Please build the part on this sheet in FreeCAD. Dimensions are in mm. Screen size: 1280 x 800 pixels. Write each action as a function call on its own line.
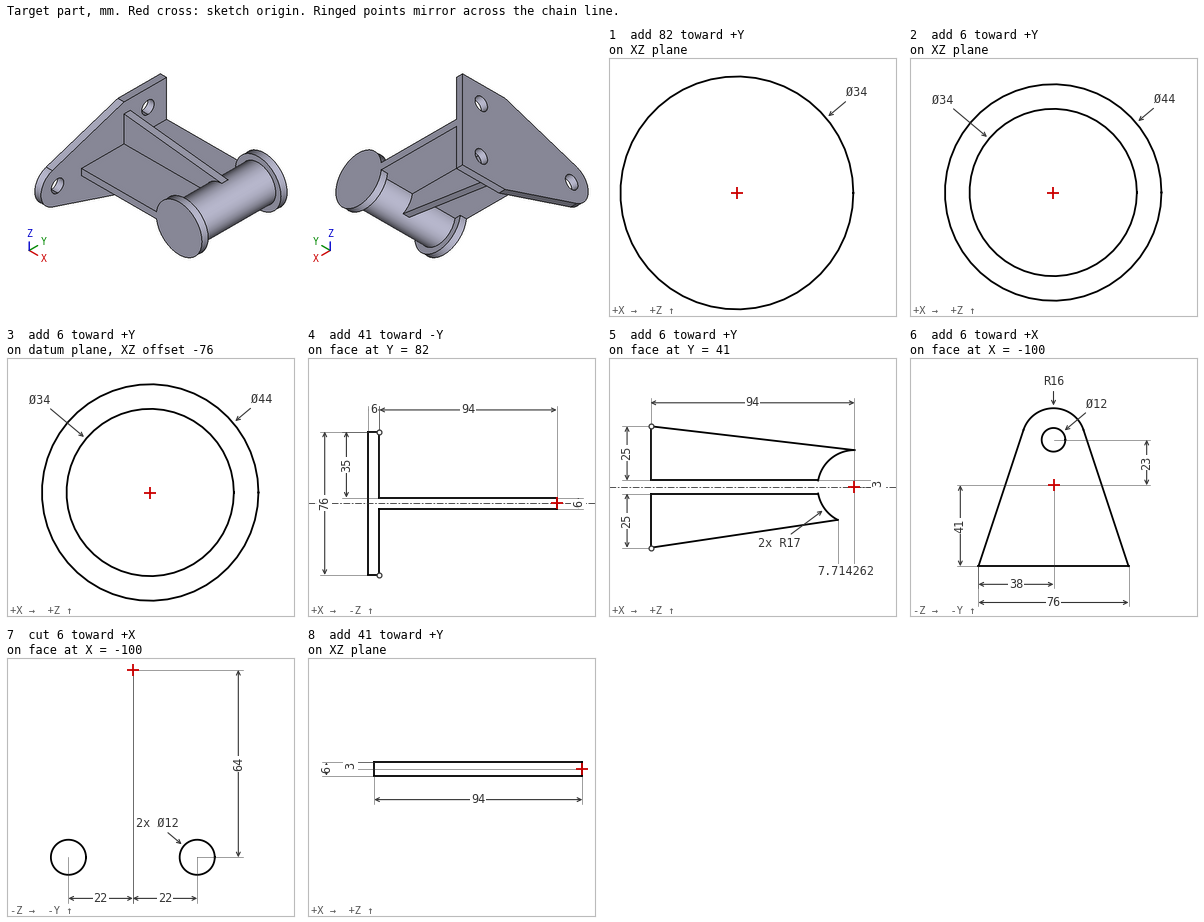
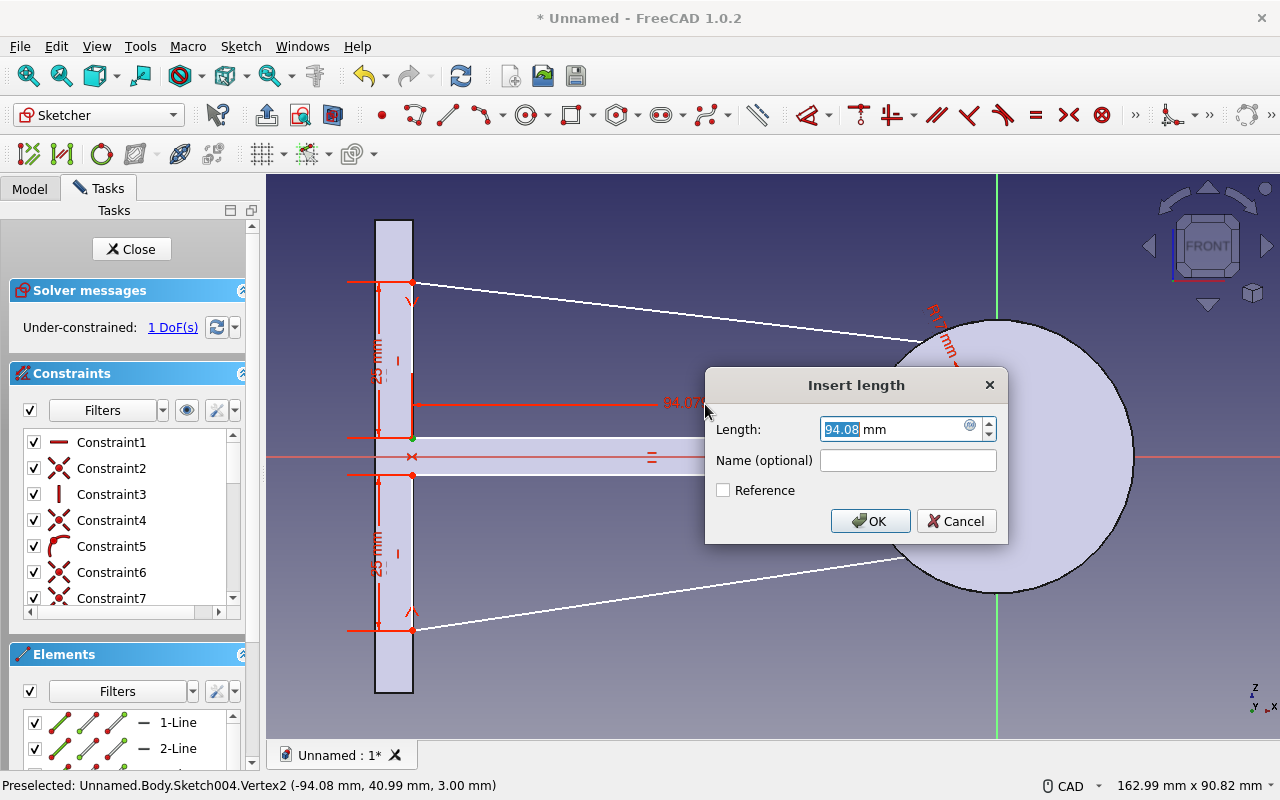
text(94)
key(Return)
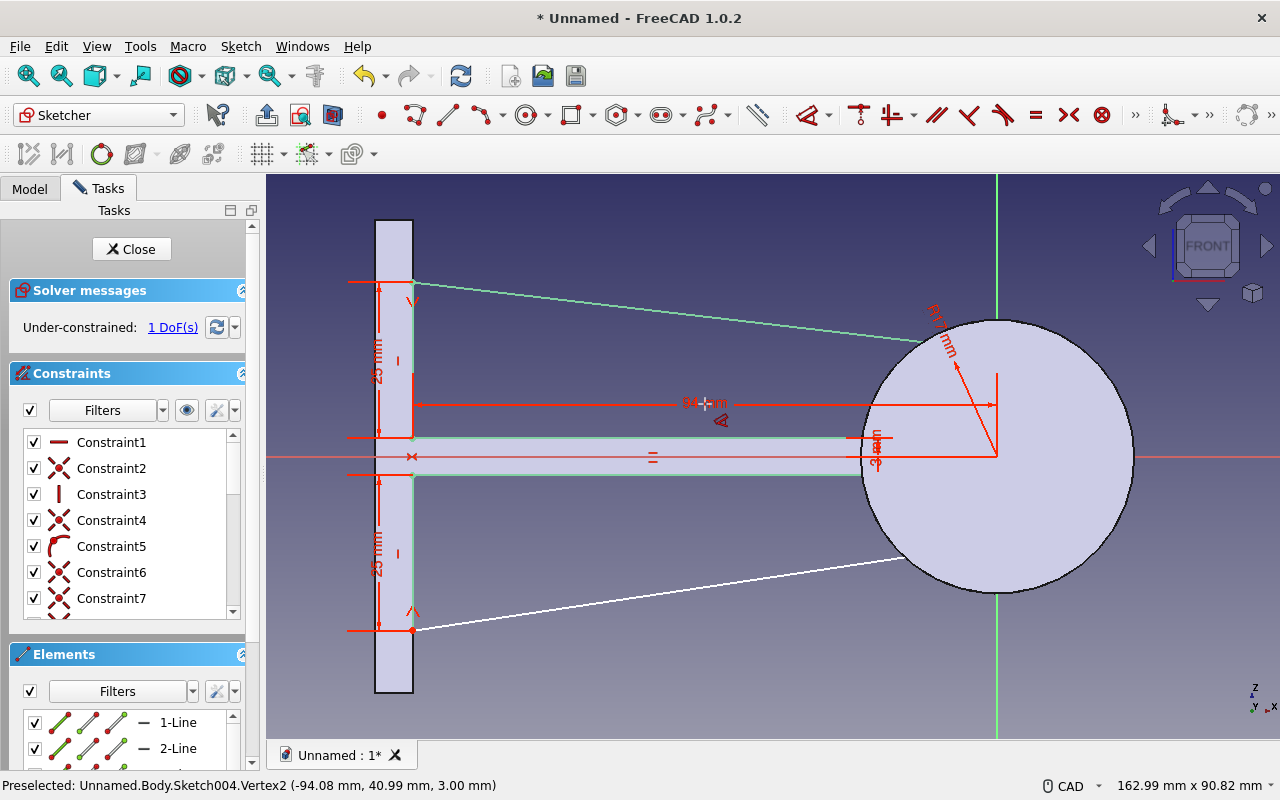
click(949, 551)
click(973, 585)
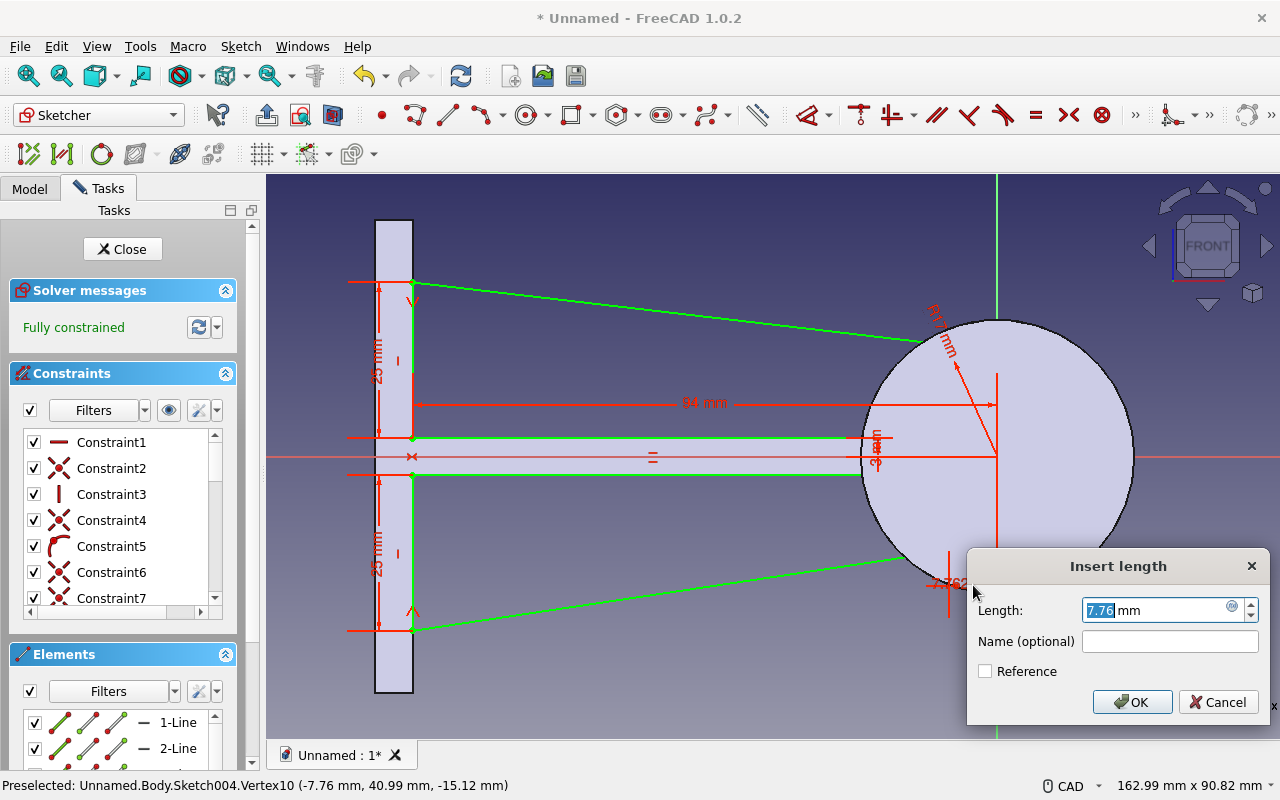
text(7.714262)
key(Return)
key(Escape)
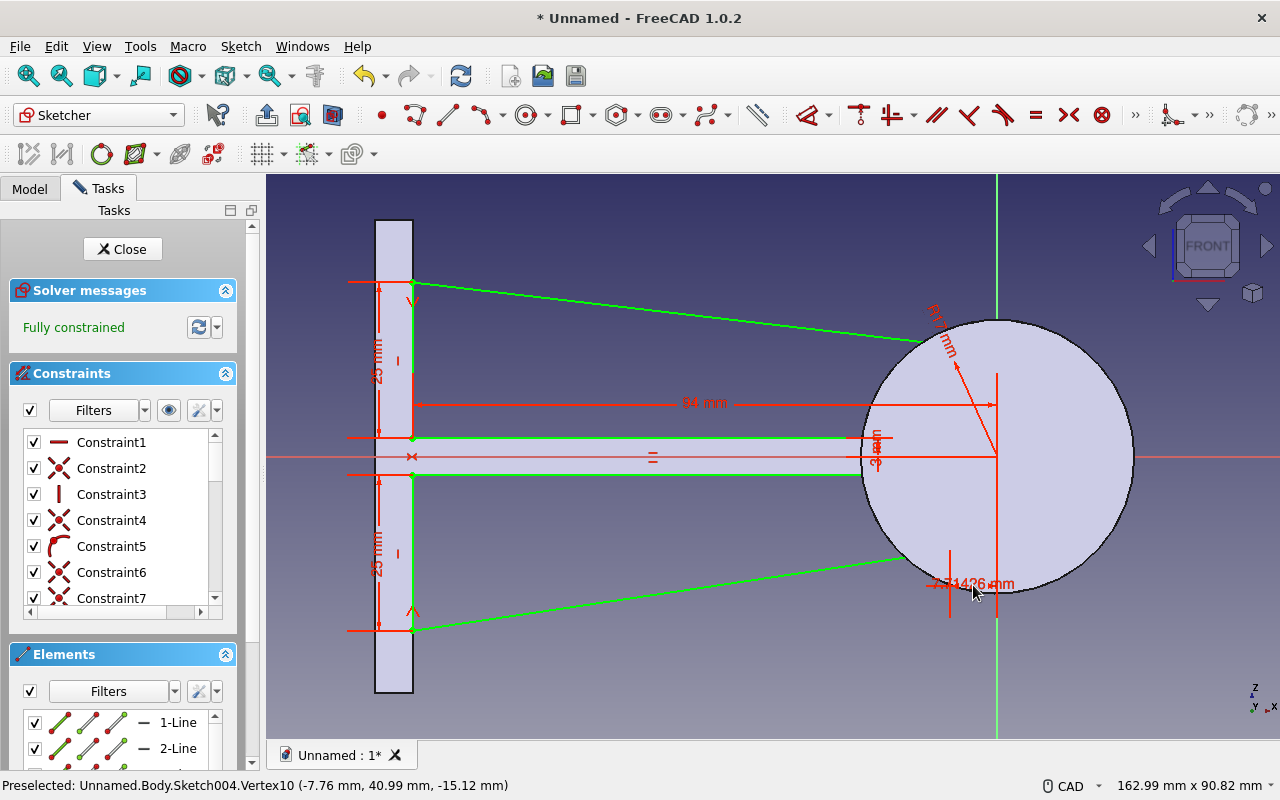
click(123, 249)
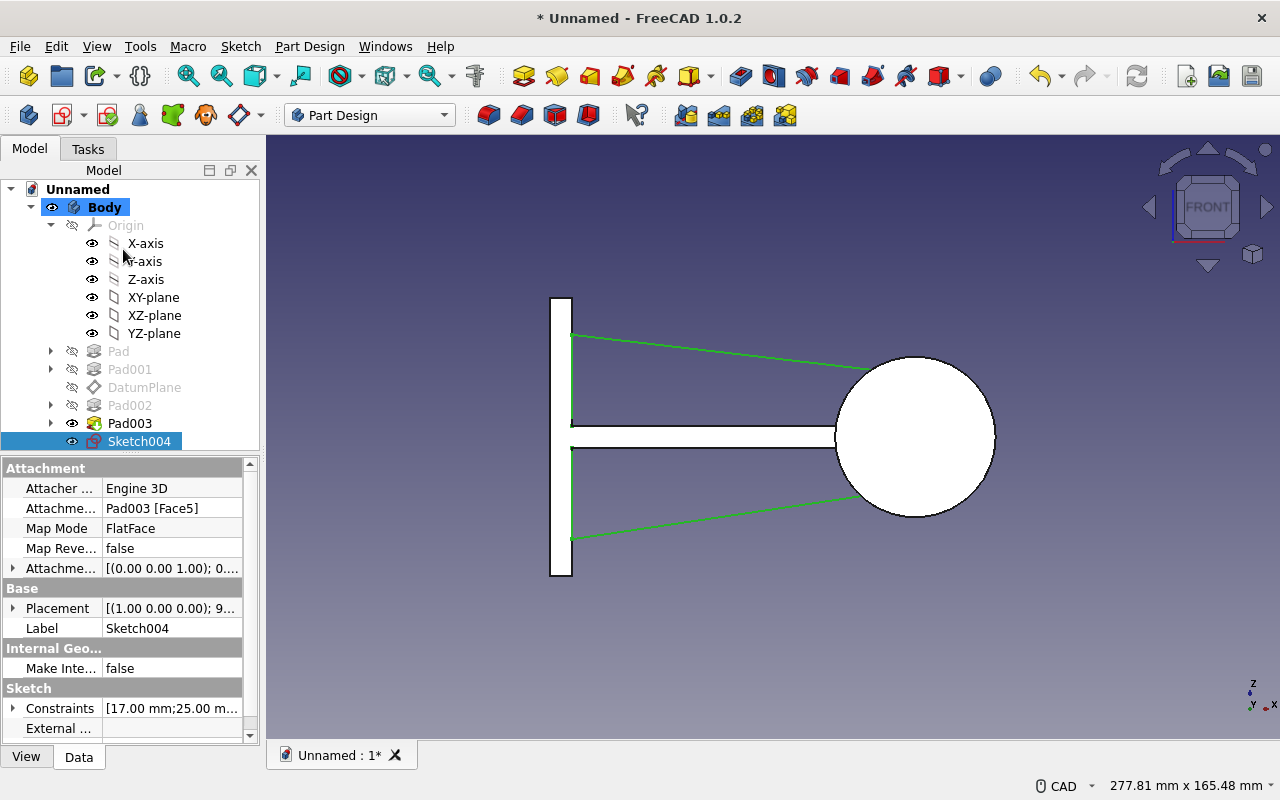
click(524, 76)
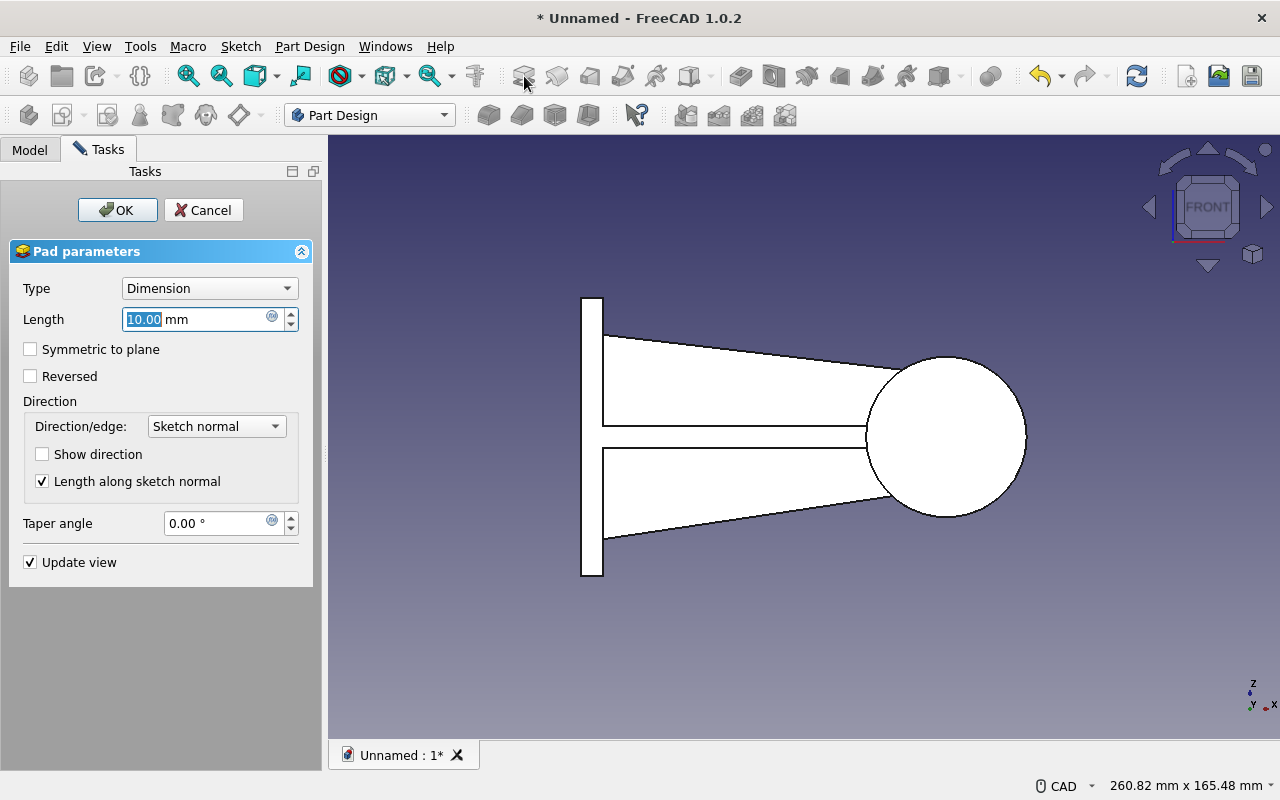
text(6)
key(Tab)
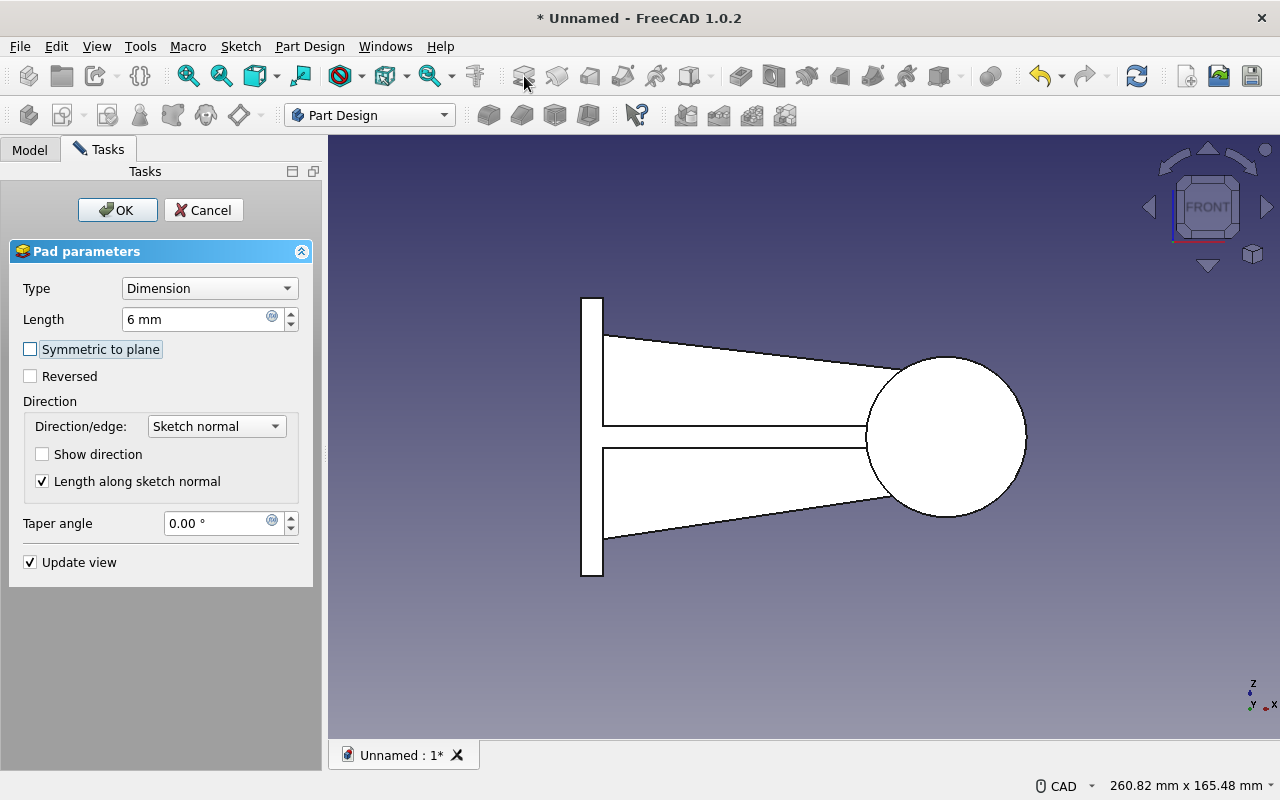
click(31, 376)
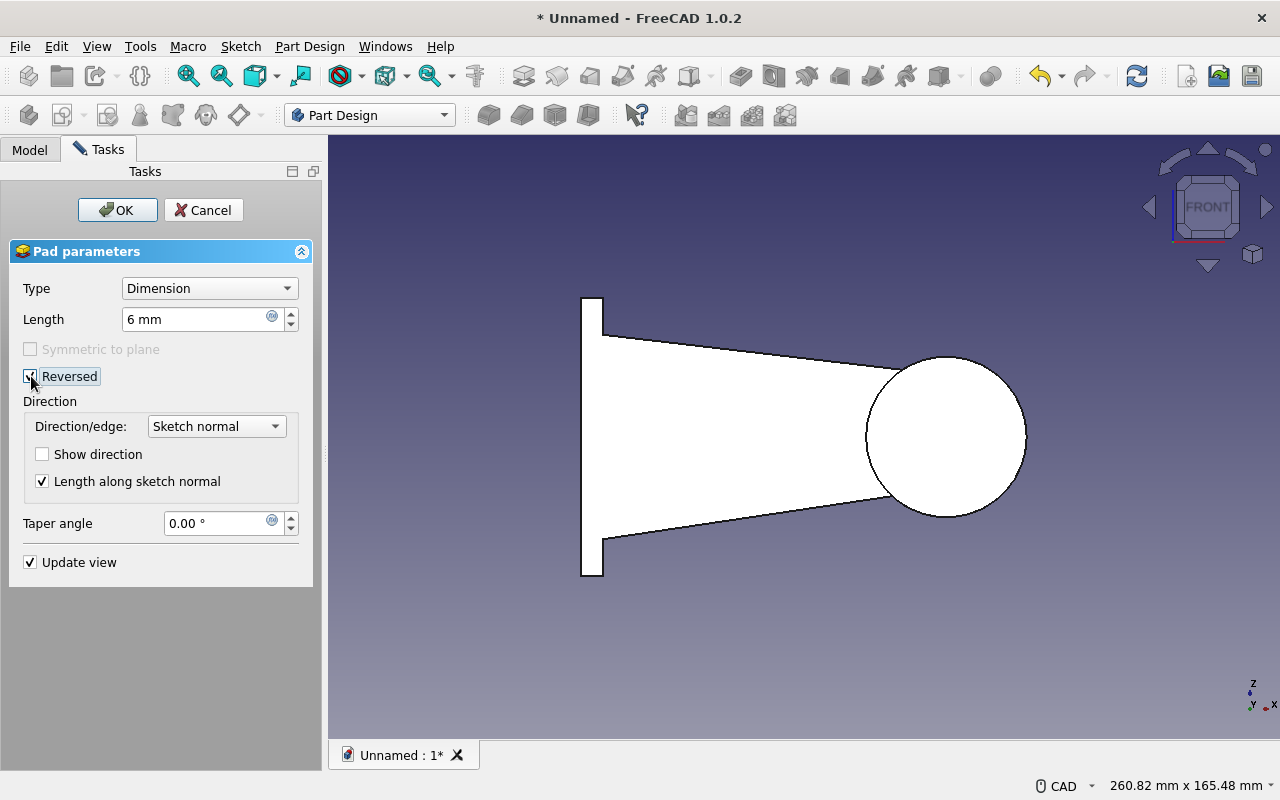
click(118, 210)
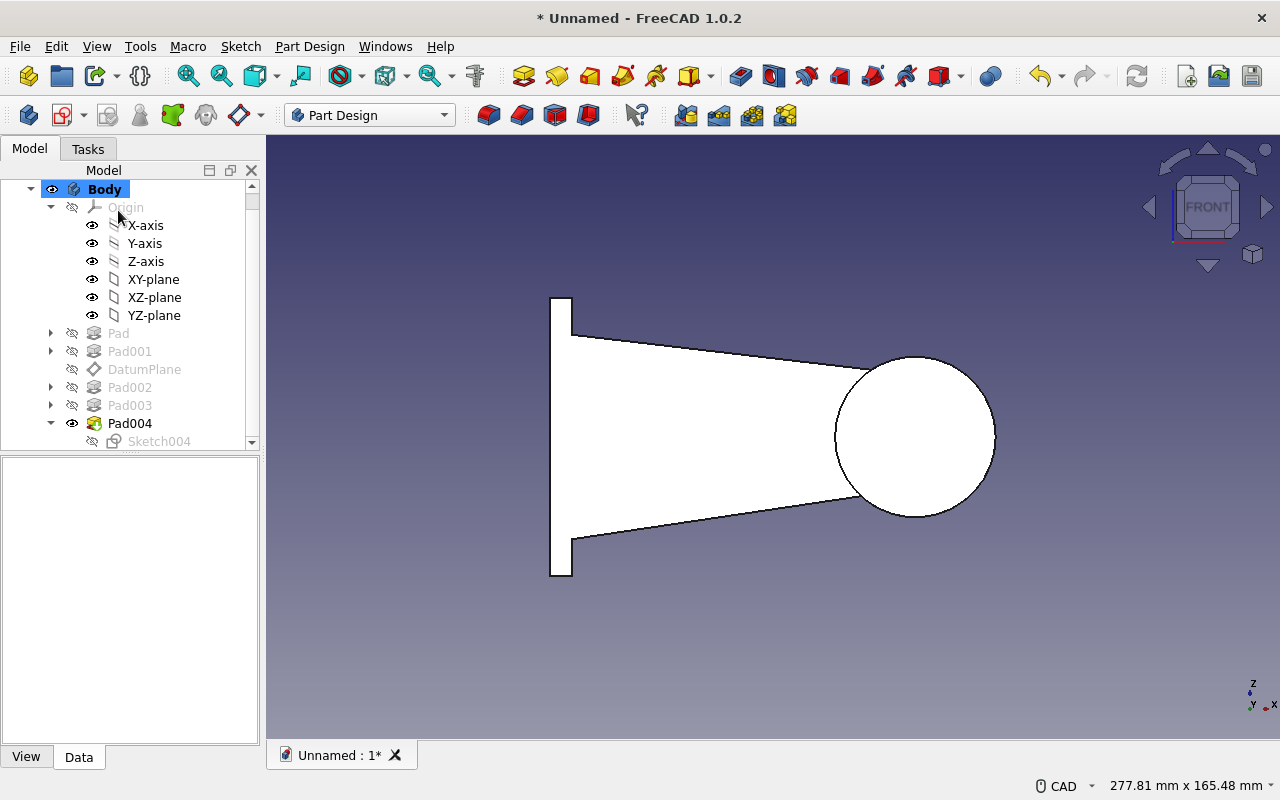
key(6)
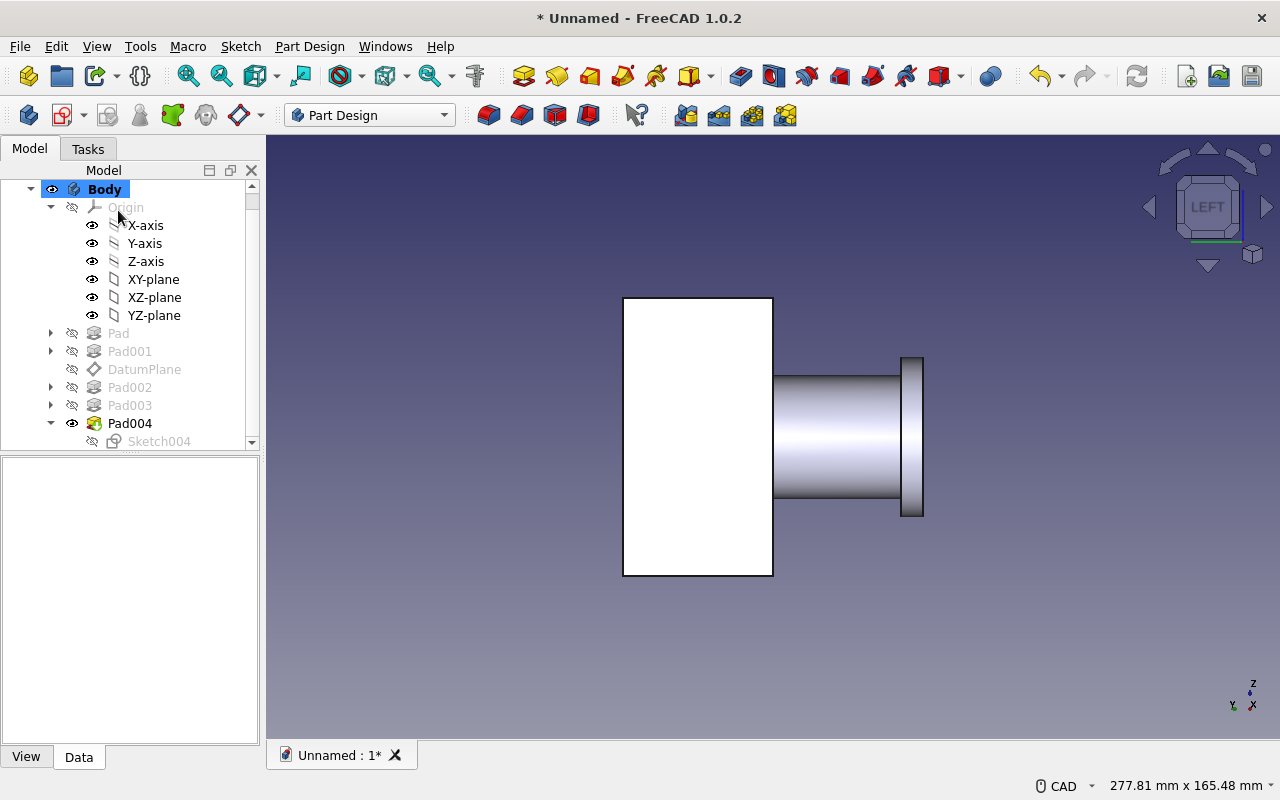
click(698, 396)